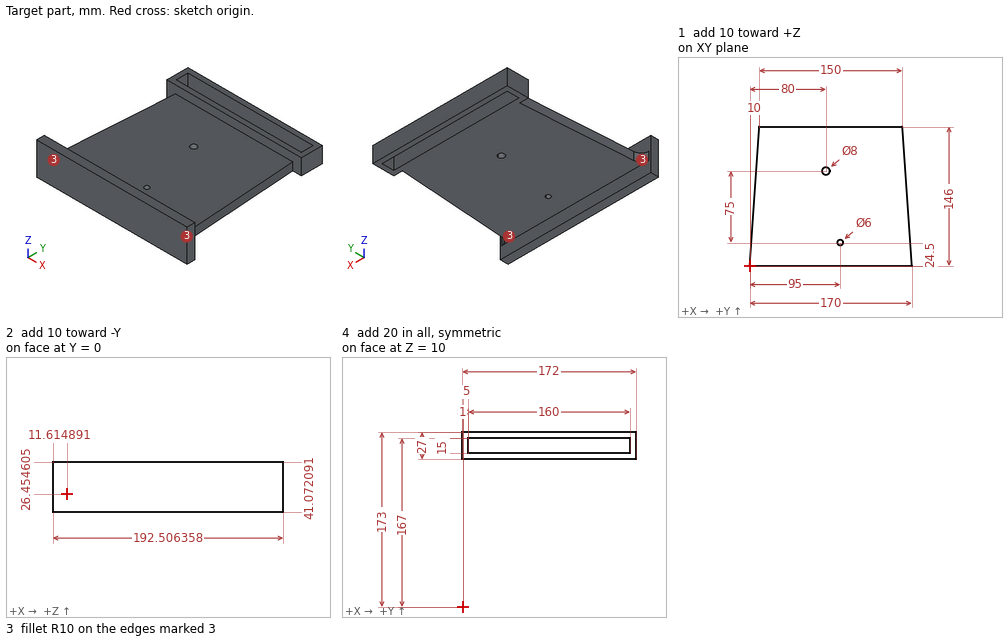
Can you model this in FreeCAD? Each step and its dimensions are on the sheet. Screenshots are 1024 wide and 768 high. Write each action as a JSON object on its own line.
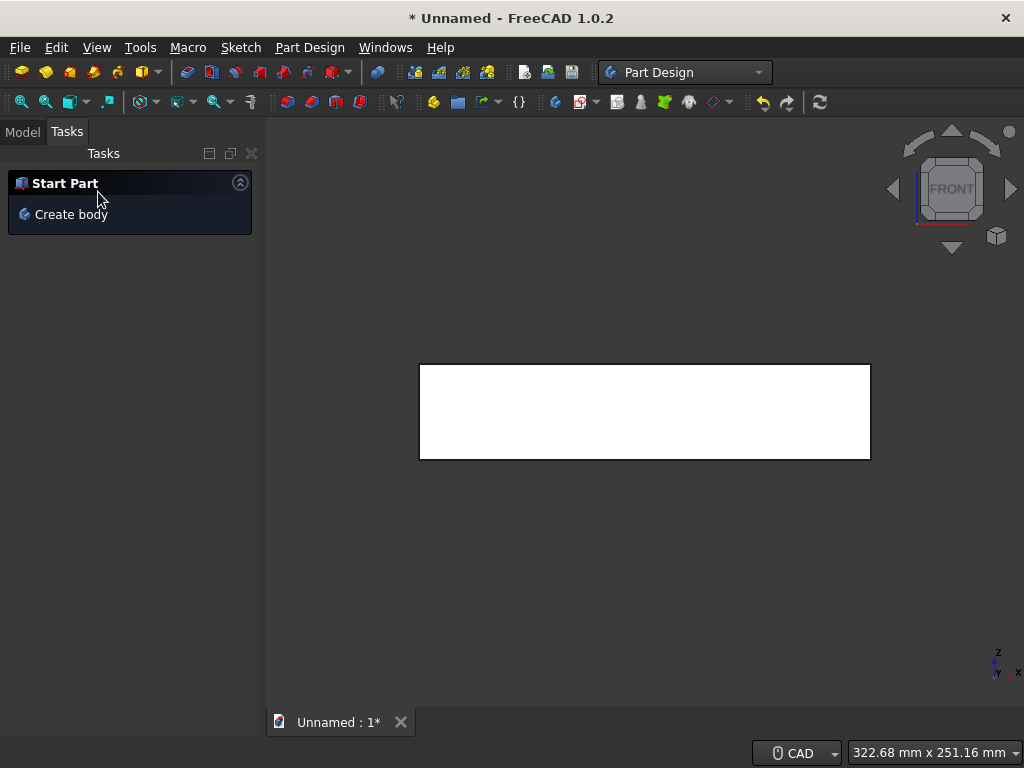
{"action": "key", "text": "0"}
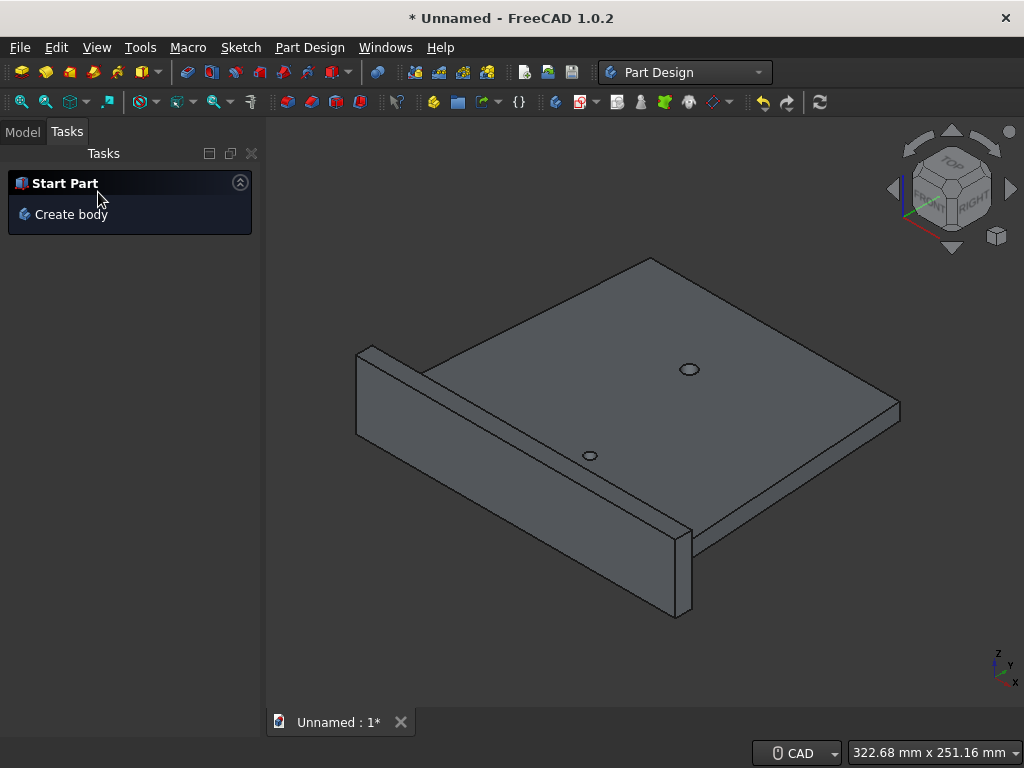
{"action": "left_click", "coordinate": [574, 393]}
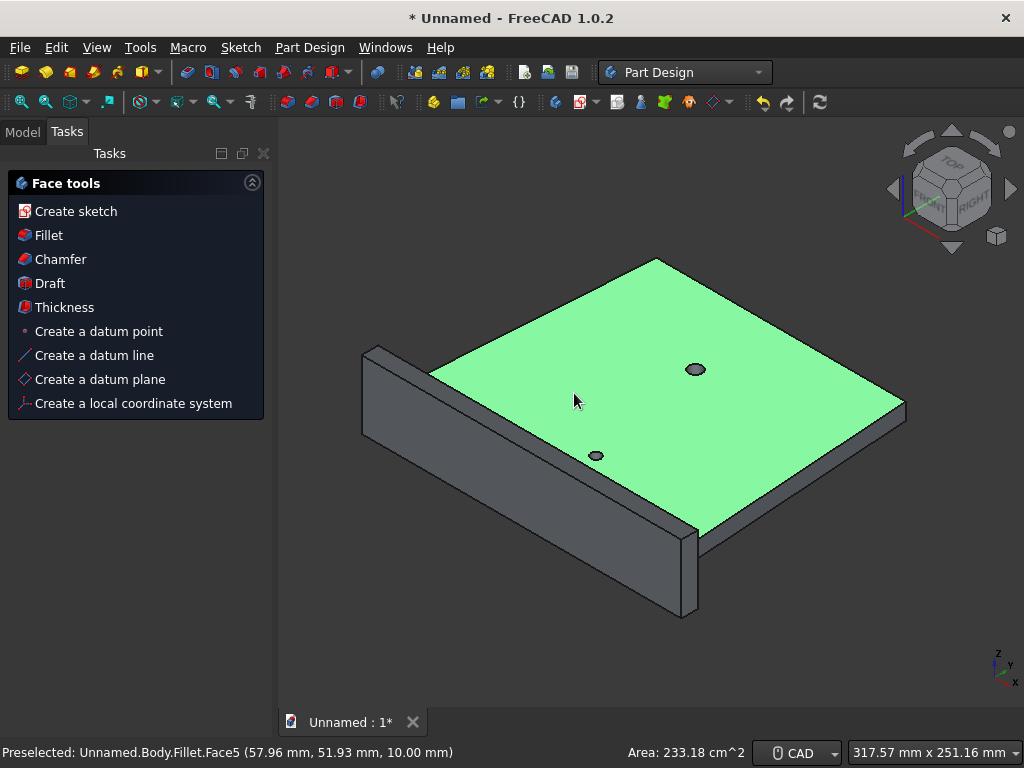
{"action": "left_click", "coordinate": [580, 102]}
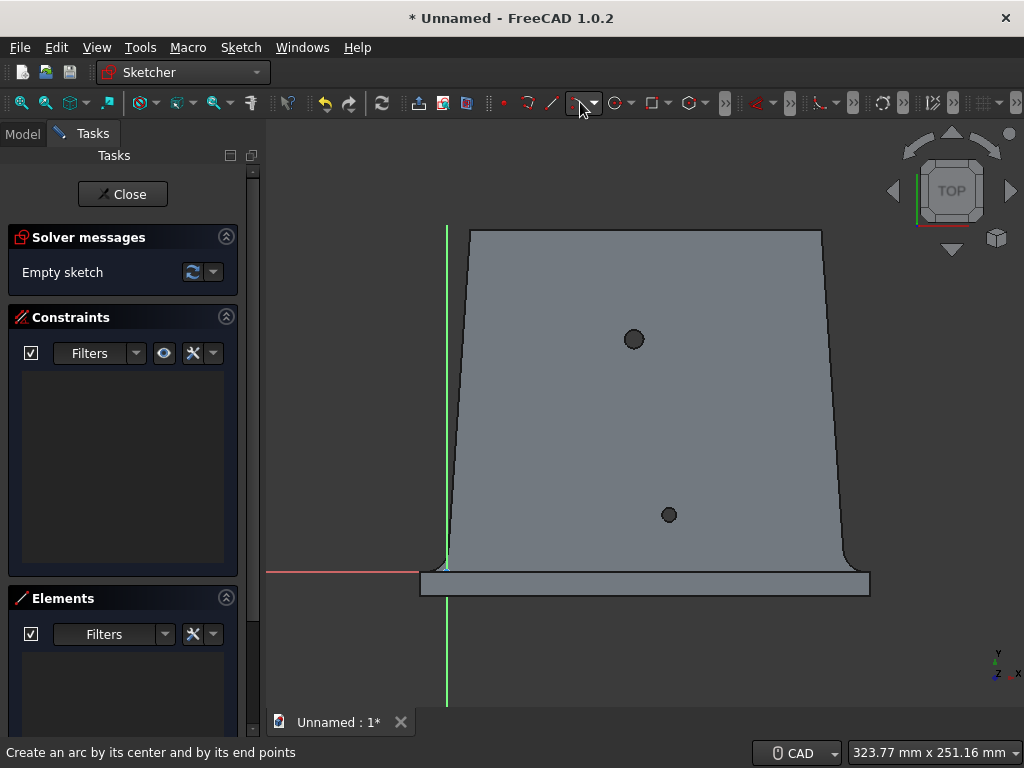
{"action": "key", "text": "q s"}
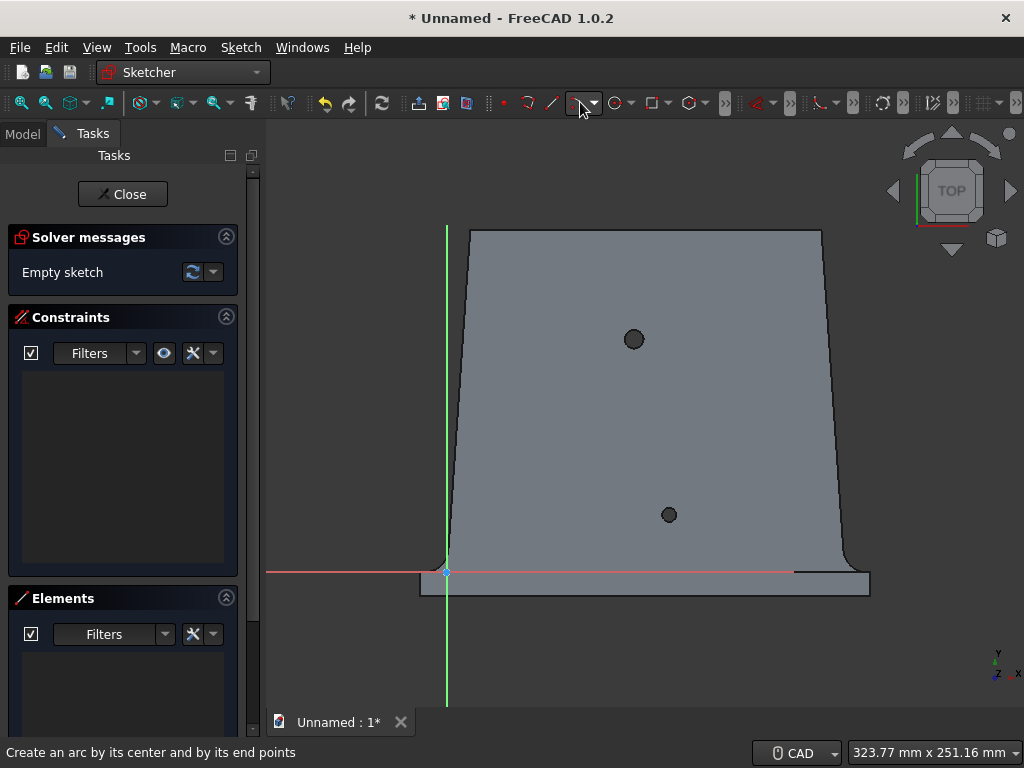
{"action": "scroll", "coordinate": [294, 609], "scroll_direction": "down", "scroll_amount": 1}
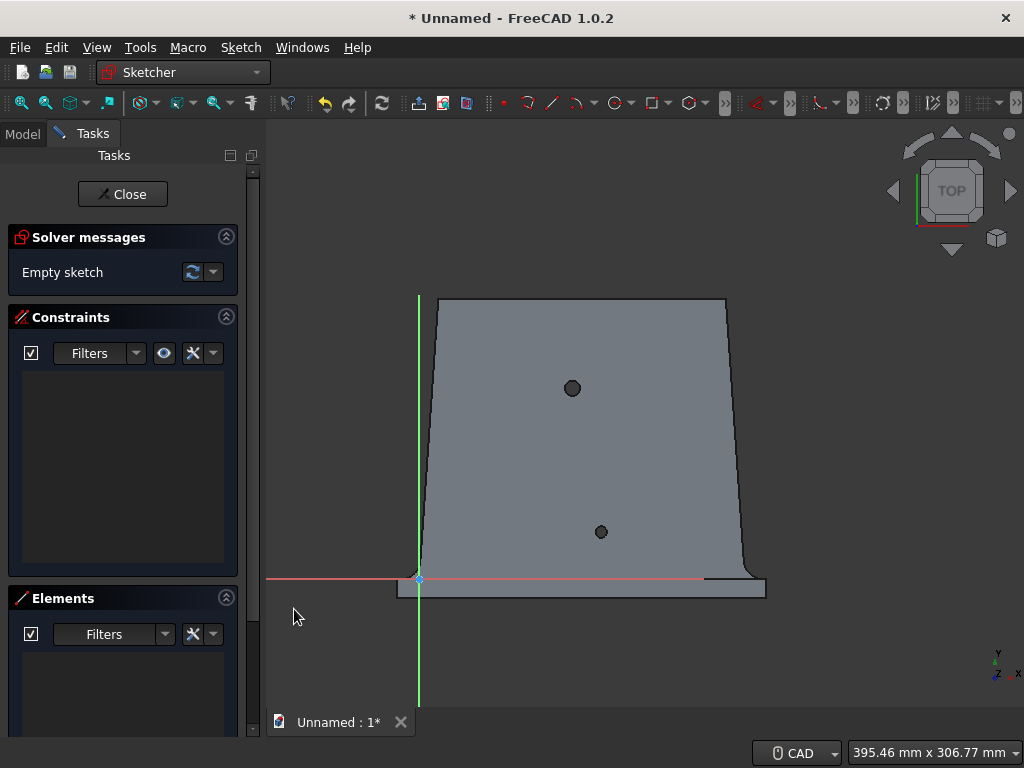
{"action": "key", "text": "g r"}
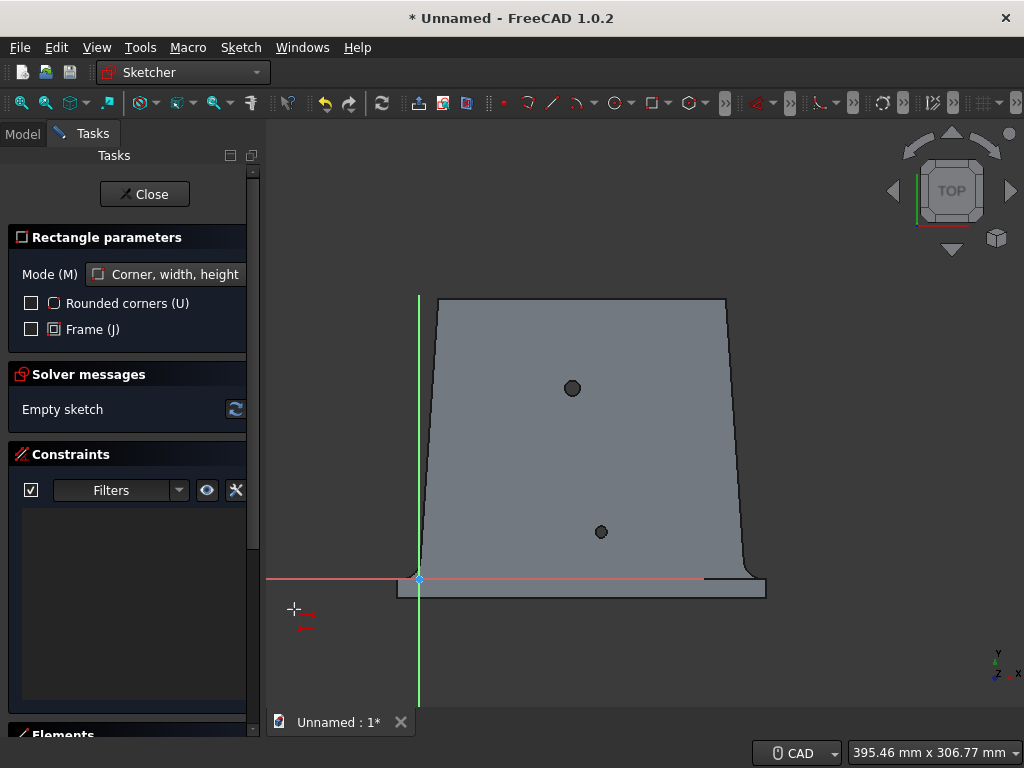
{"action": "scroll", "coordinate": [417, 247], "scroll_direction": "up", "scroll_amount": 11}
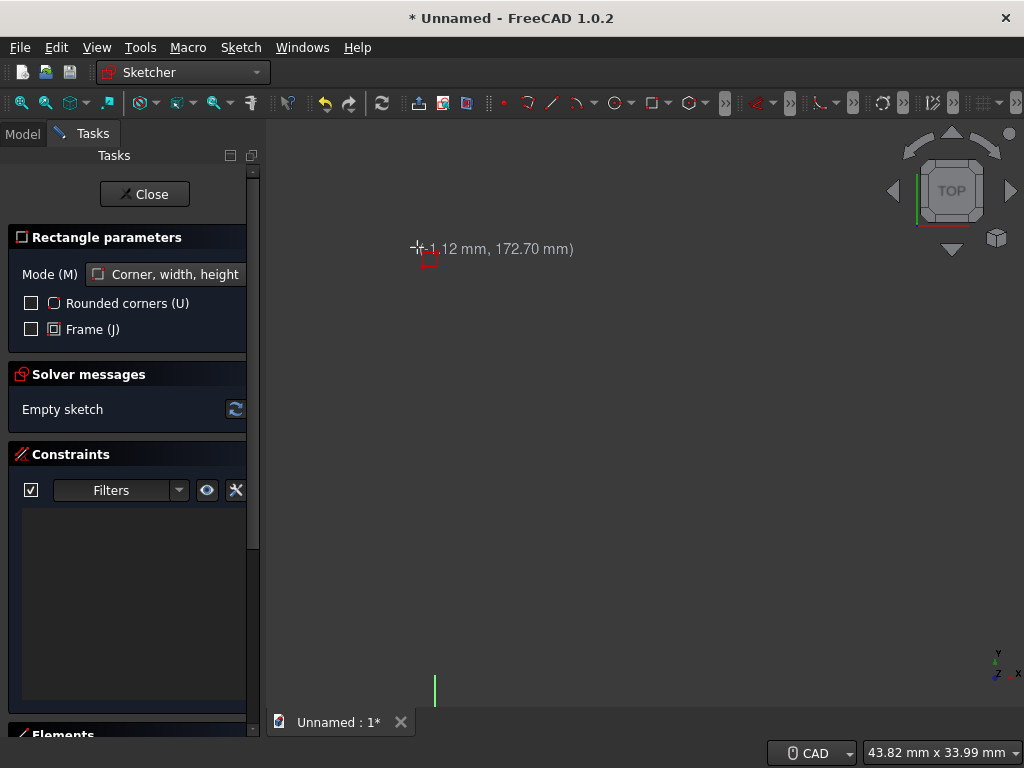
{"action": "left_click", "coordinate": [418, 249]}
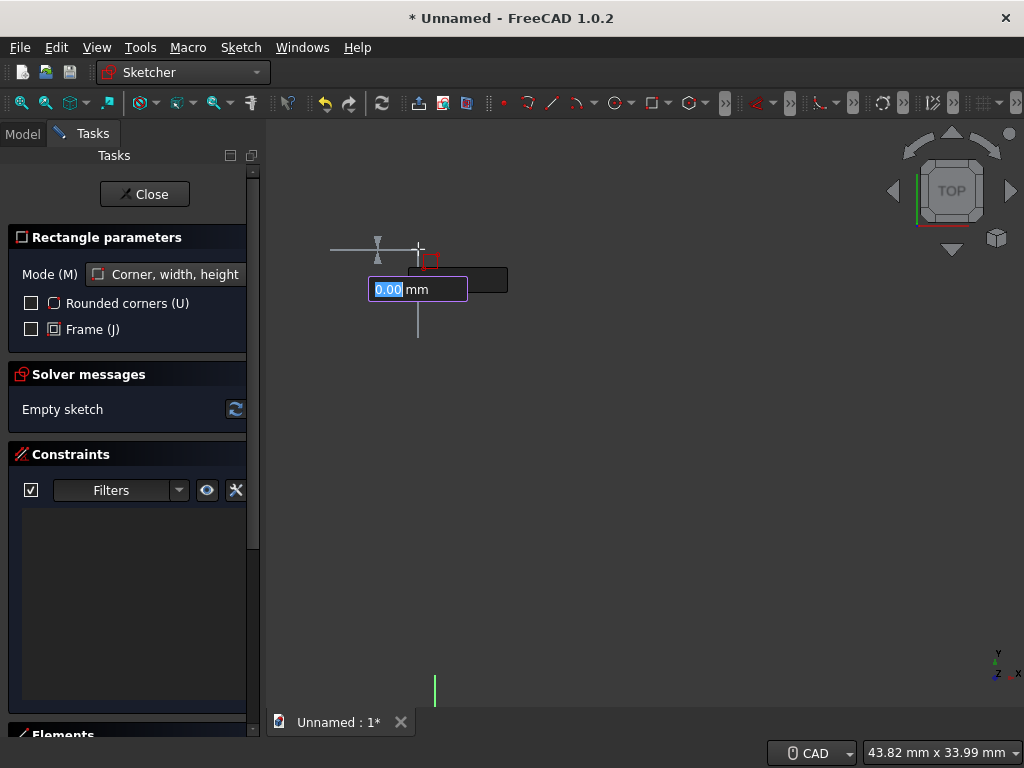
{"action": "scroll", "coordinate": [369, 204], "scroll_direction": "down", "scroll_amount": 10}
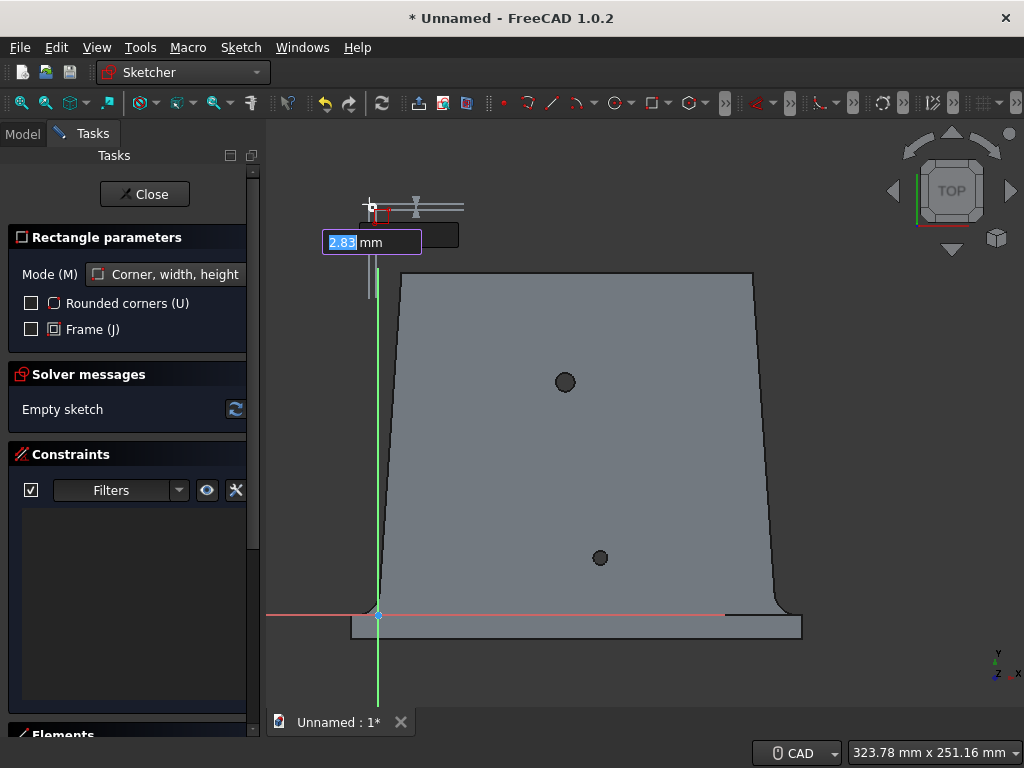
{"action": "left_click", "coordinate": [778, 273]}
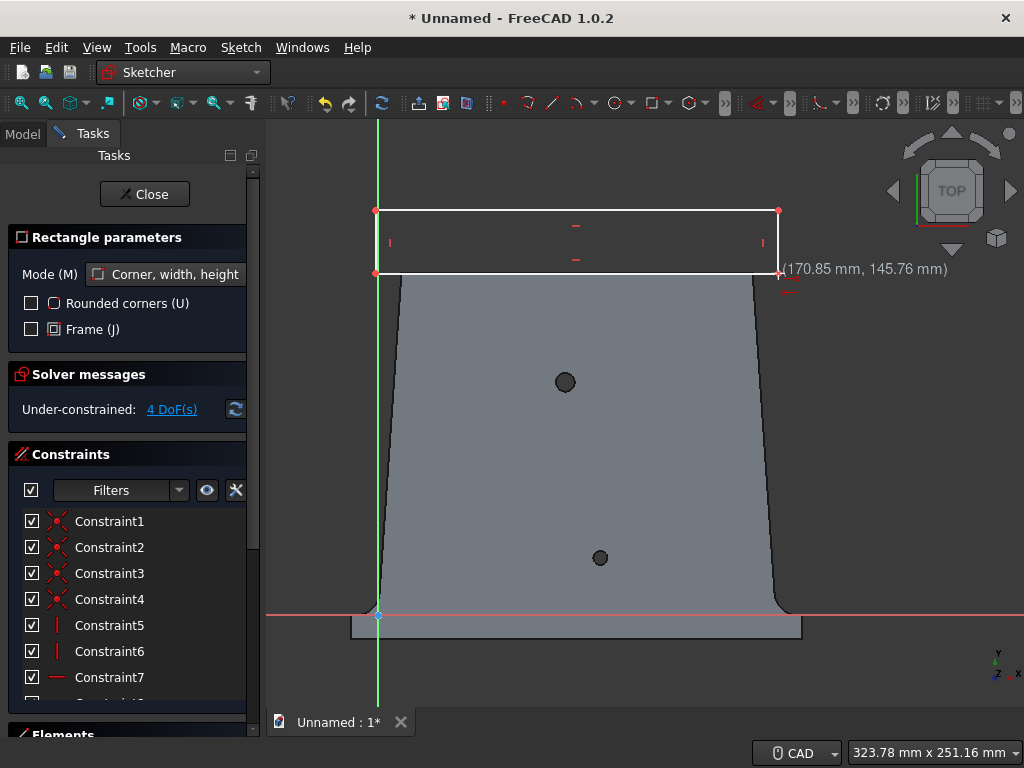
{"action": "scroll", "coordinate": [390, 224], "scroll_direction": "up", "scroll_amount": 2}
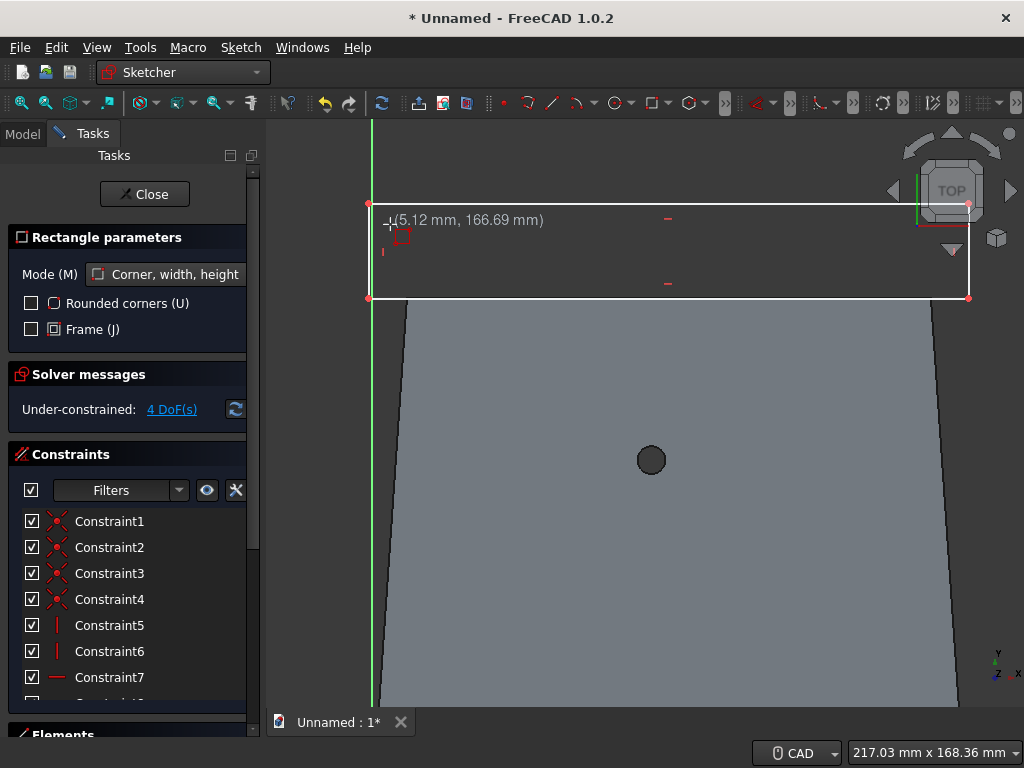
{"action": "left_click", "coordinate": [390, 224]}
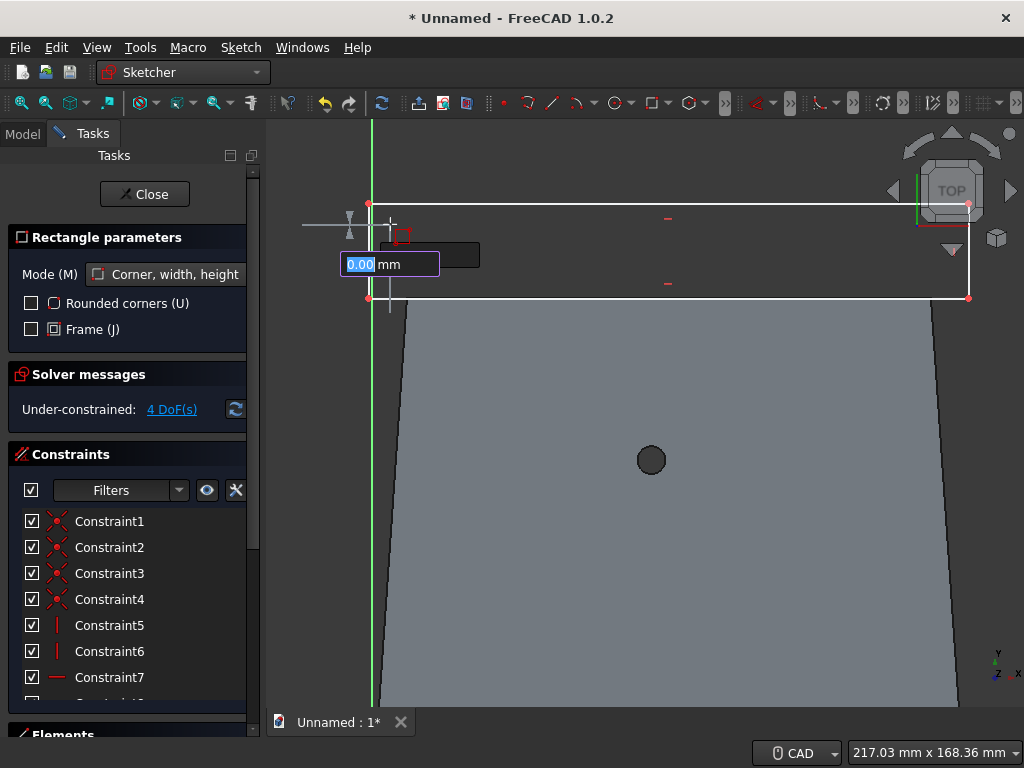
{"action": "scroll", "coordinate": [389, 225], "scroll_direction": "down", "scroll_amount": 2}